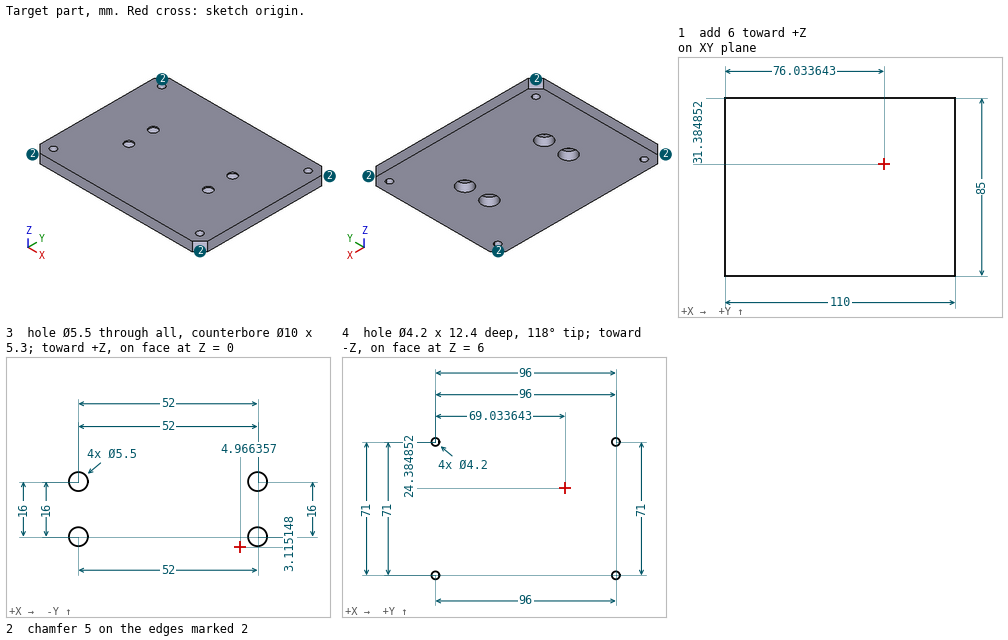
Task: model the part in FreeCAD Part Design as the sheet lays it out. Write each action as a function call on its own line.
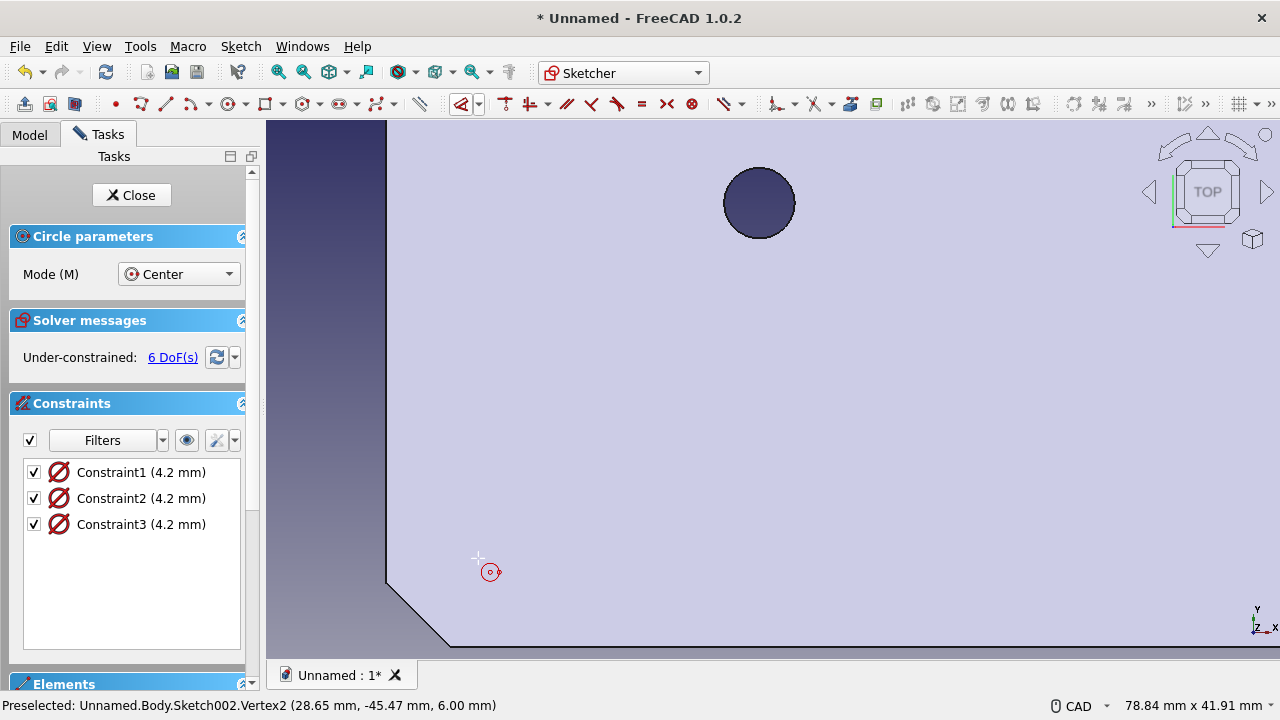
click(476, 557)
move(495, 538)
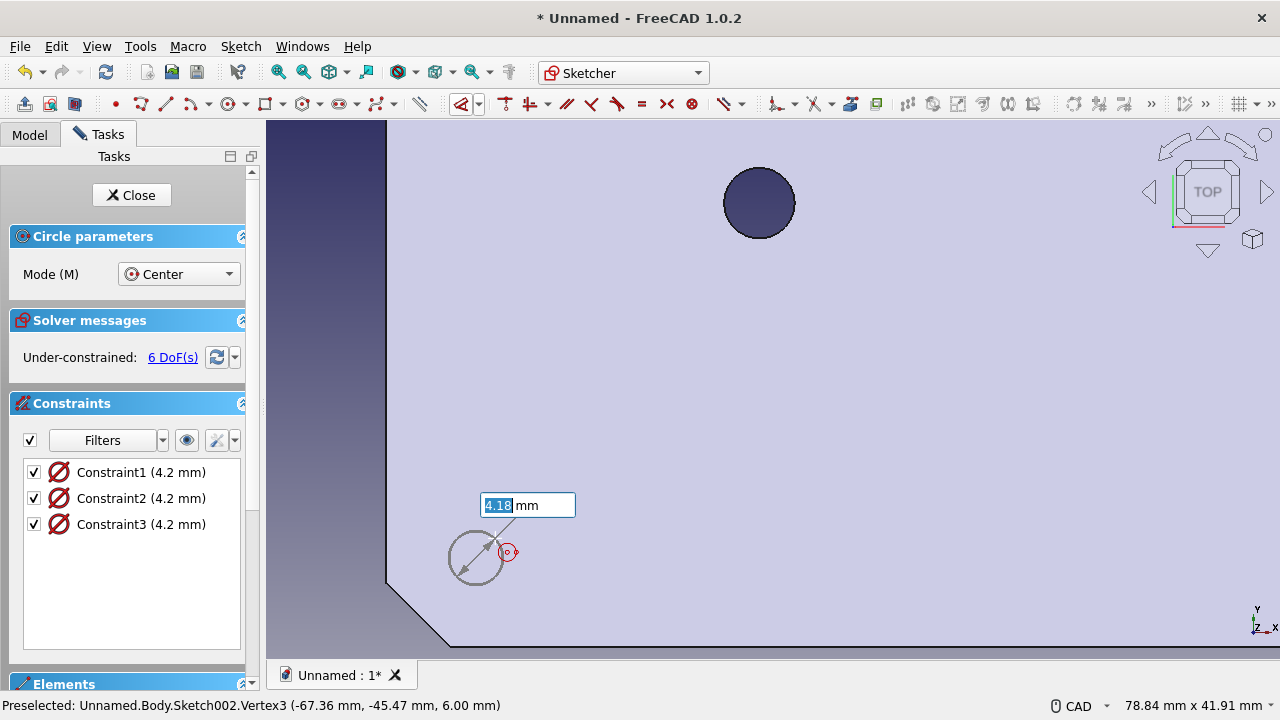
text(4.2)
key(Return)
key(Escape)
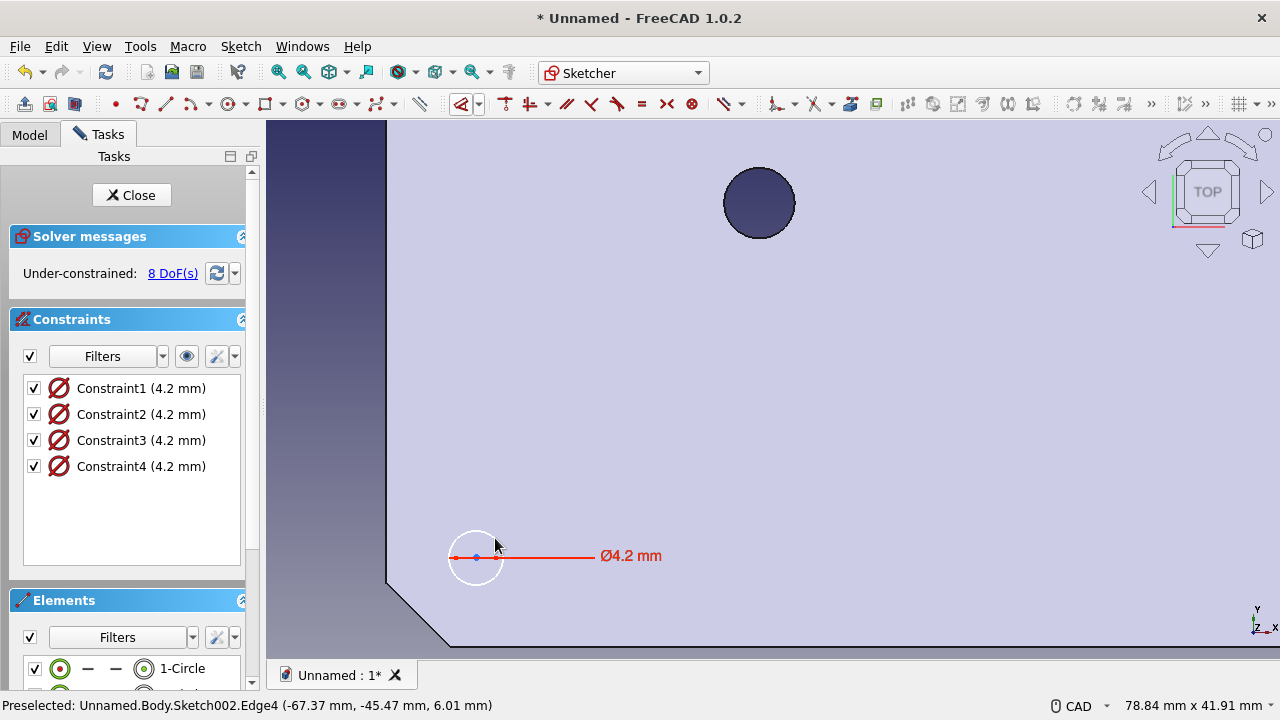
scroll(478, 558, down, 5)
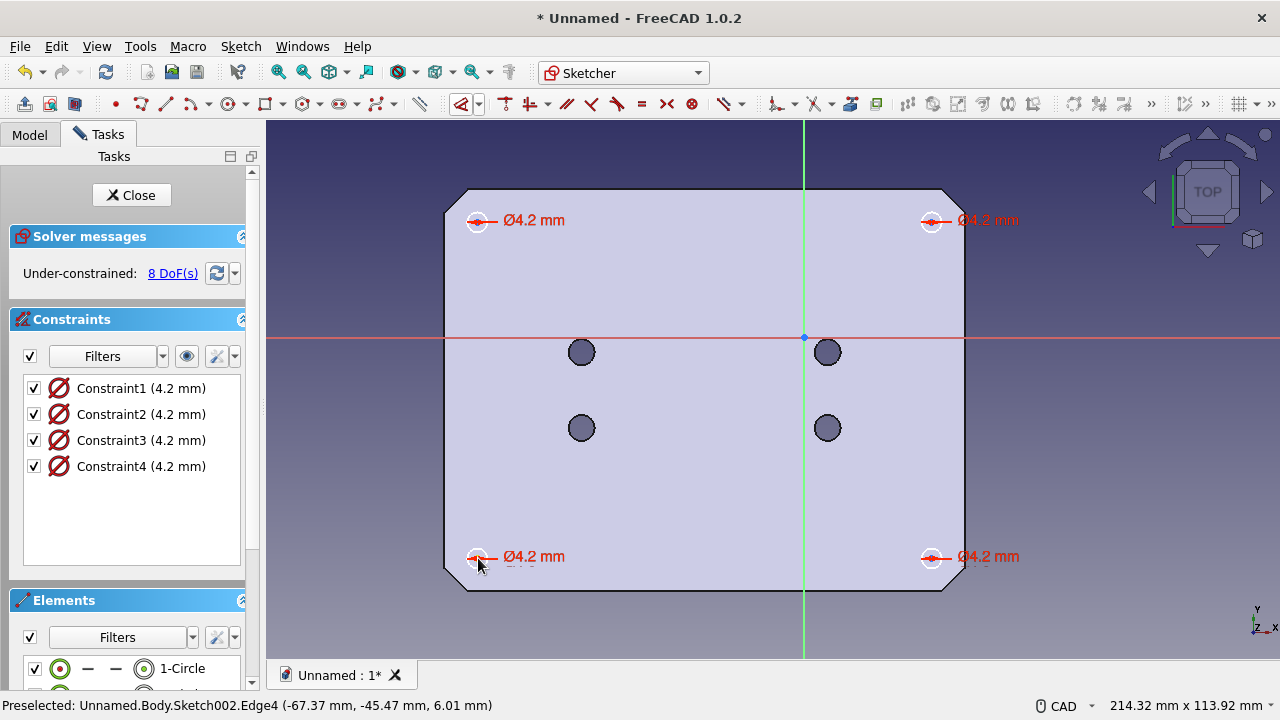
click(477, 222)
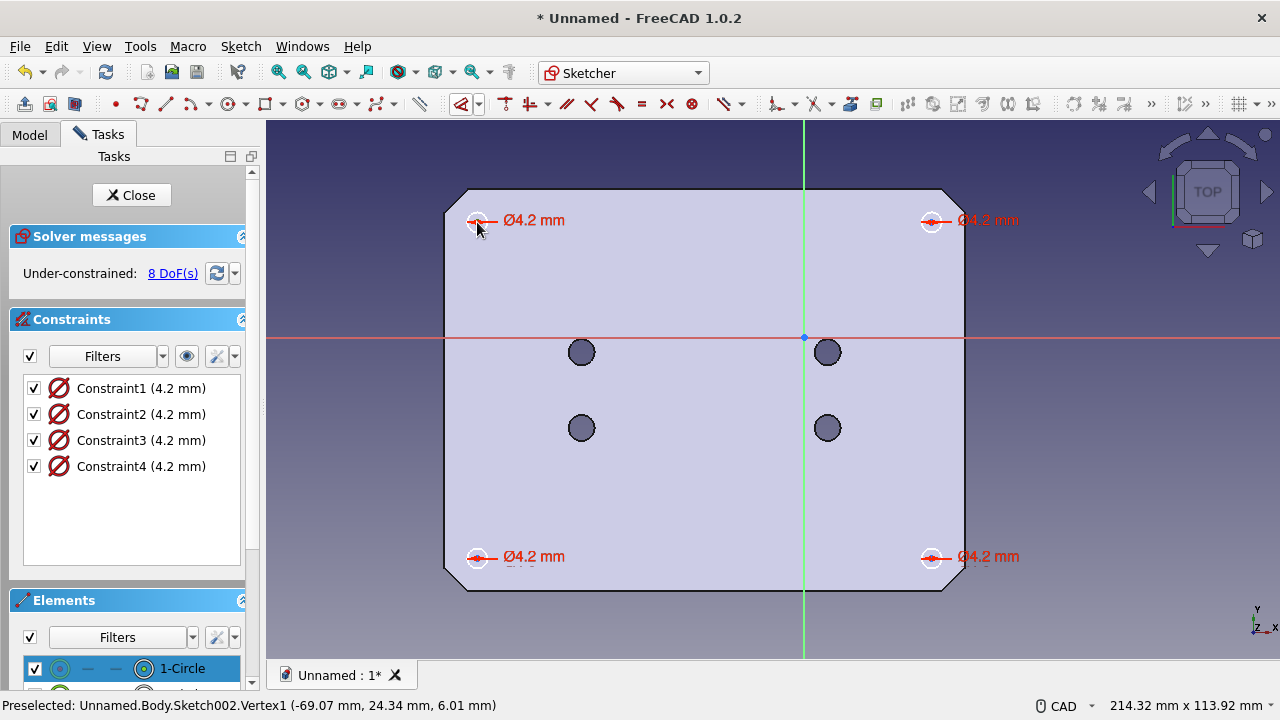
click(932, 222)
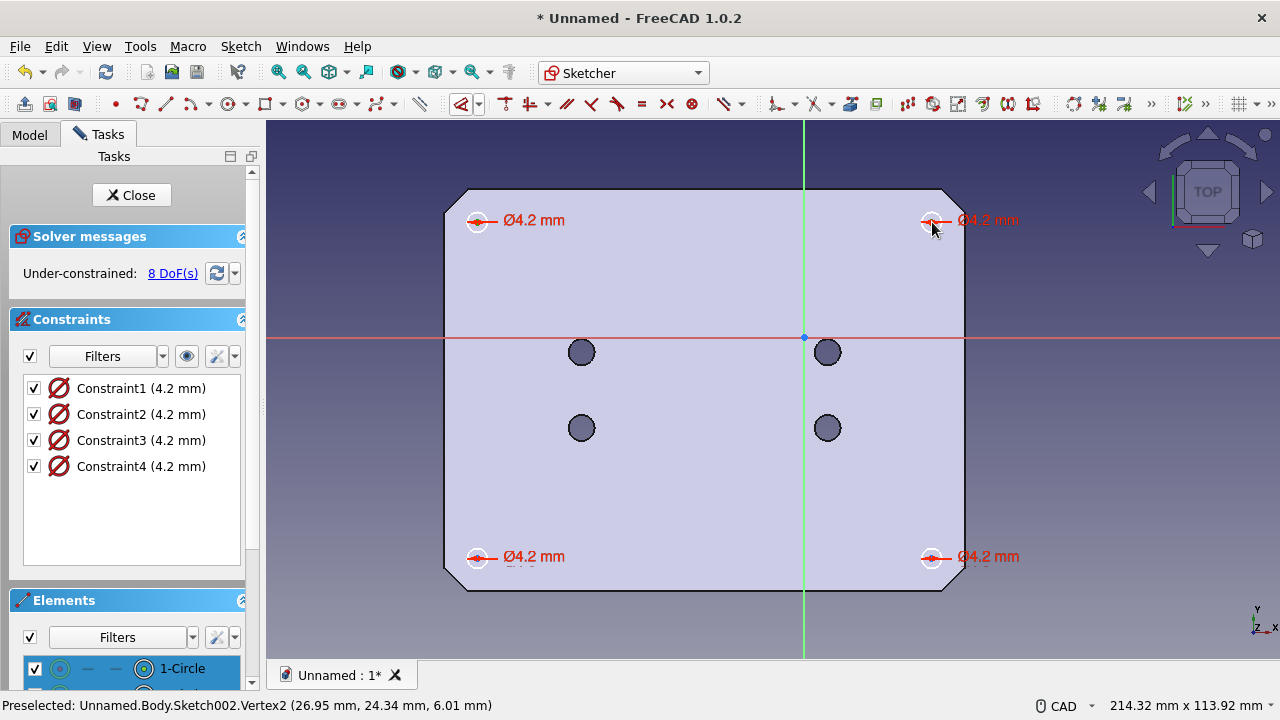
key(l)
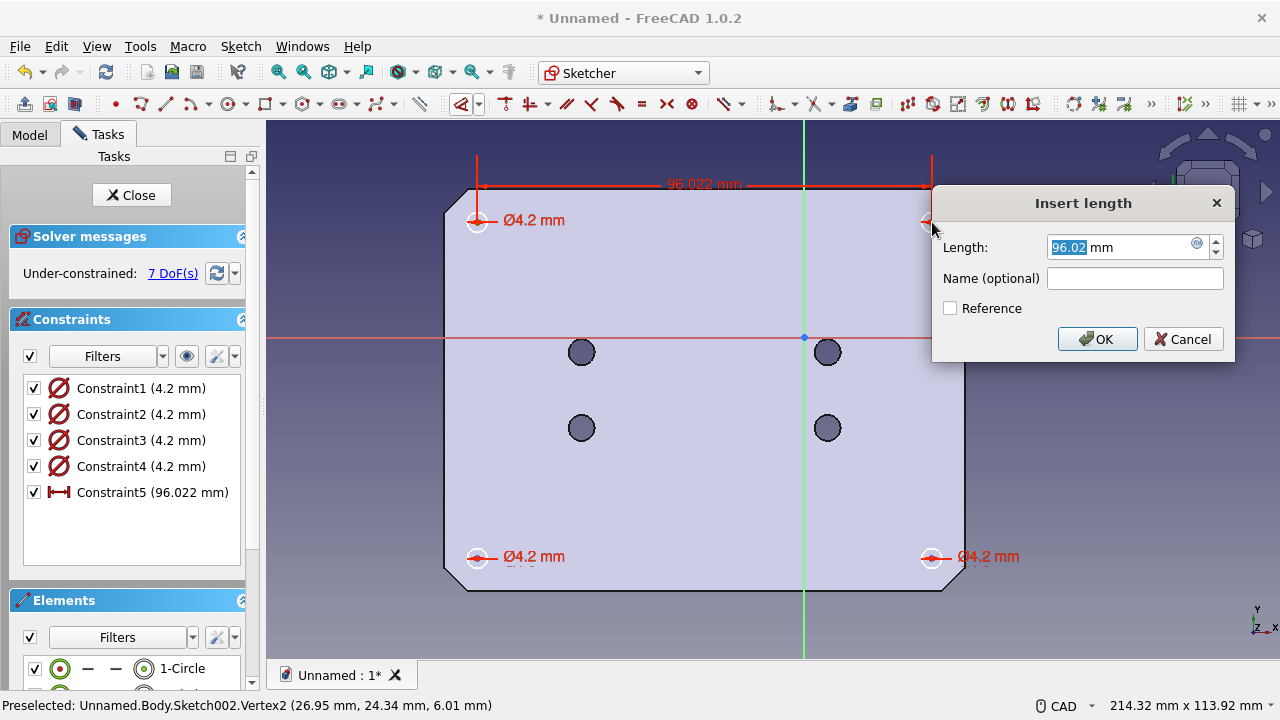
text(96)
key(Return)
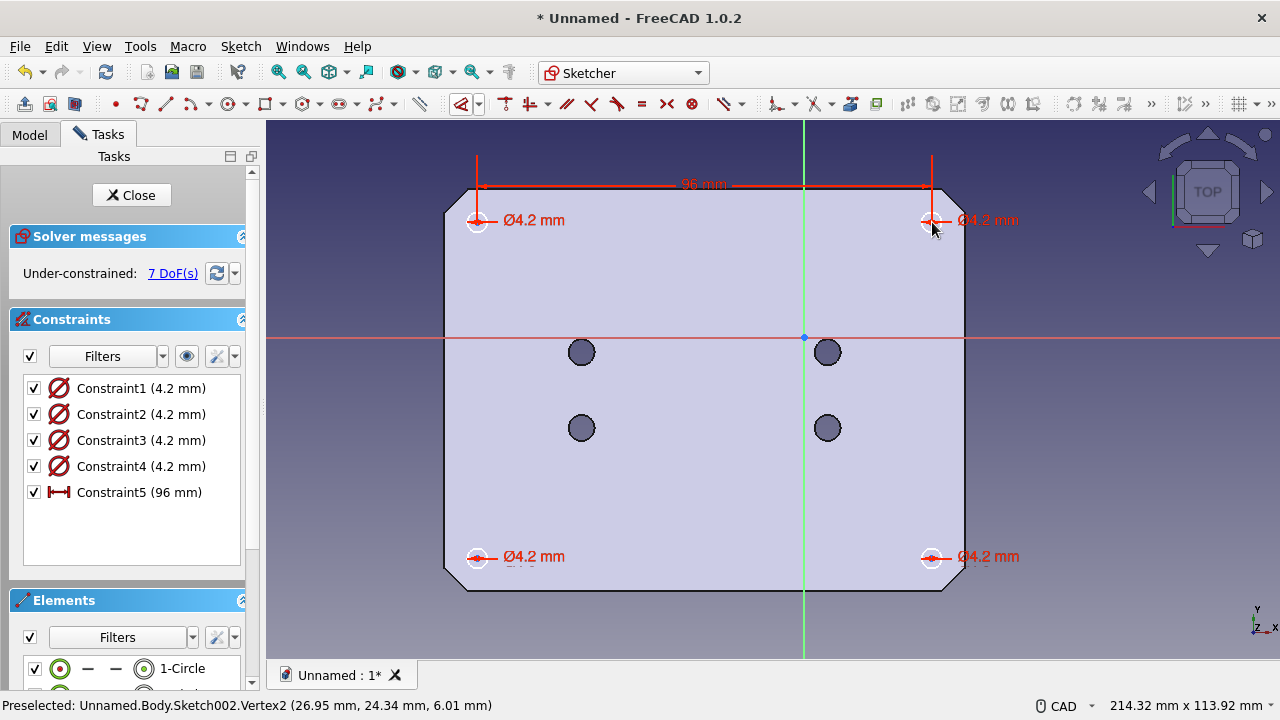
click(477, 222)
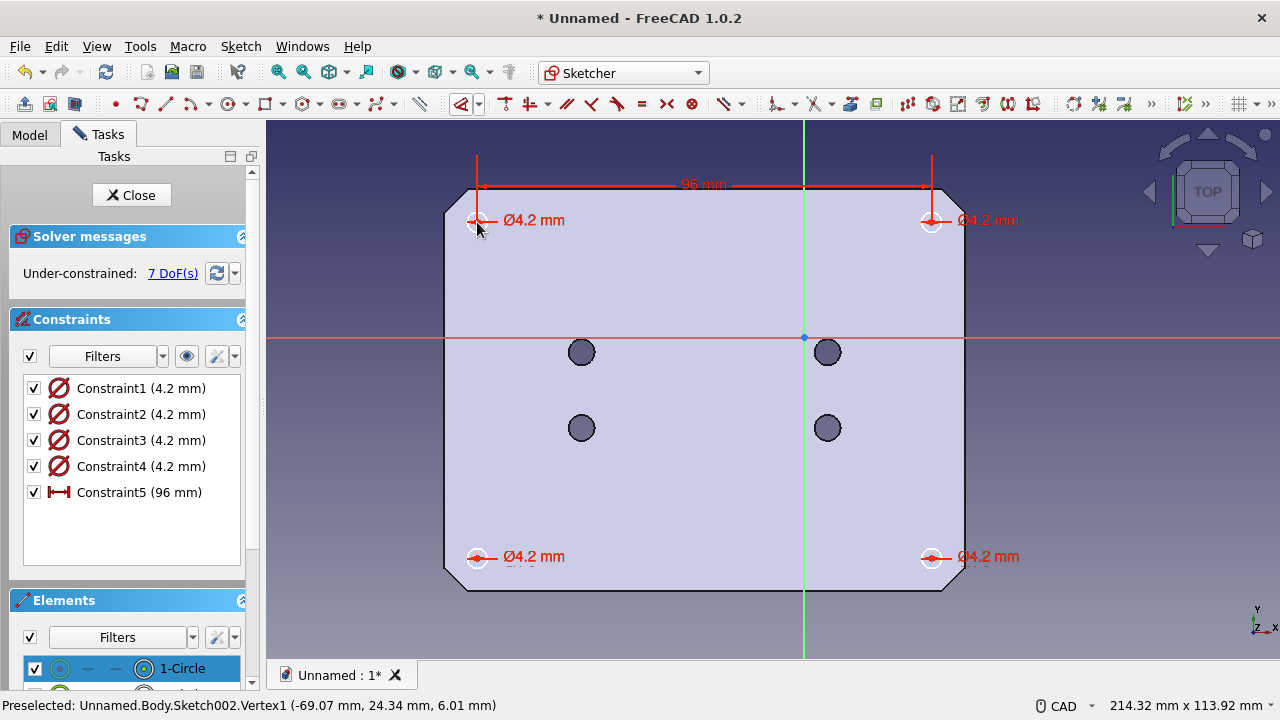
click(932, 559)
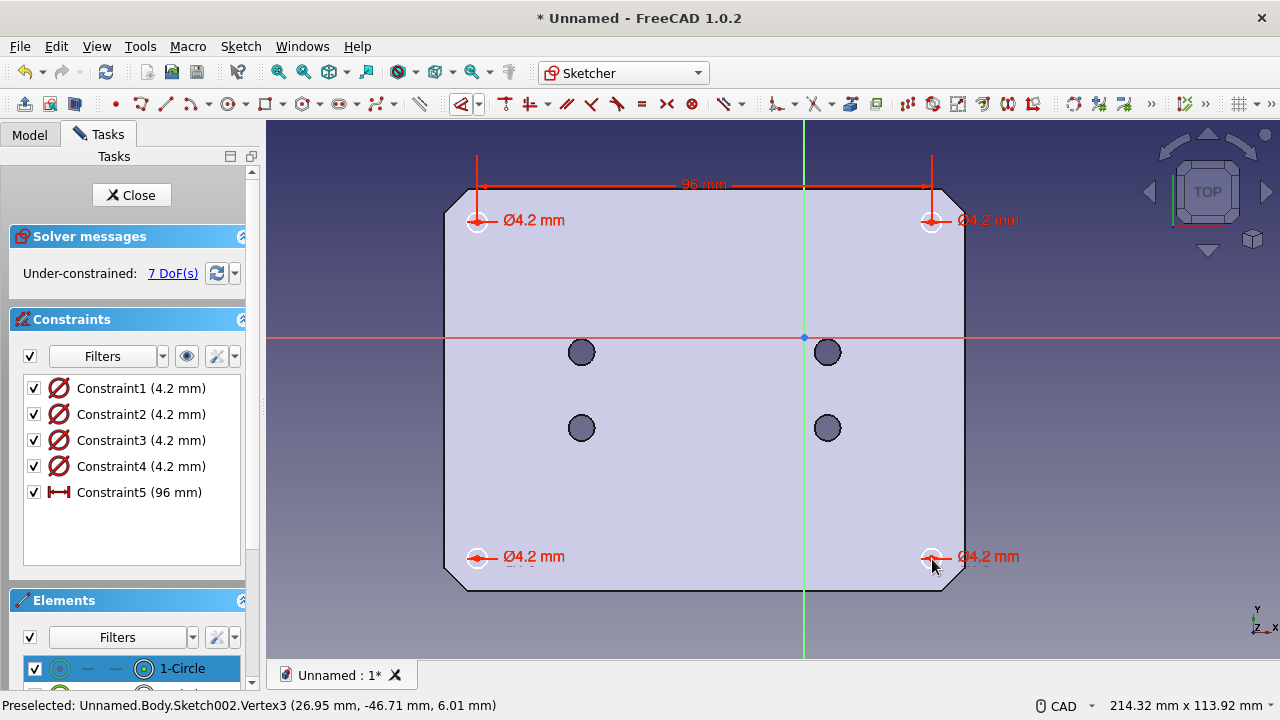
key(l)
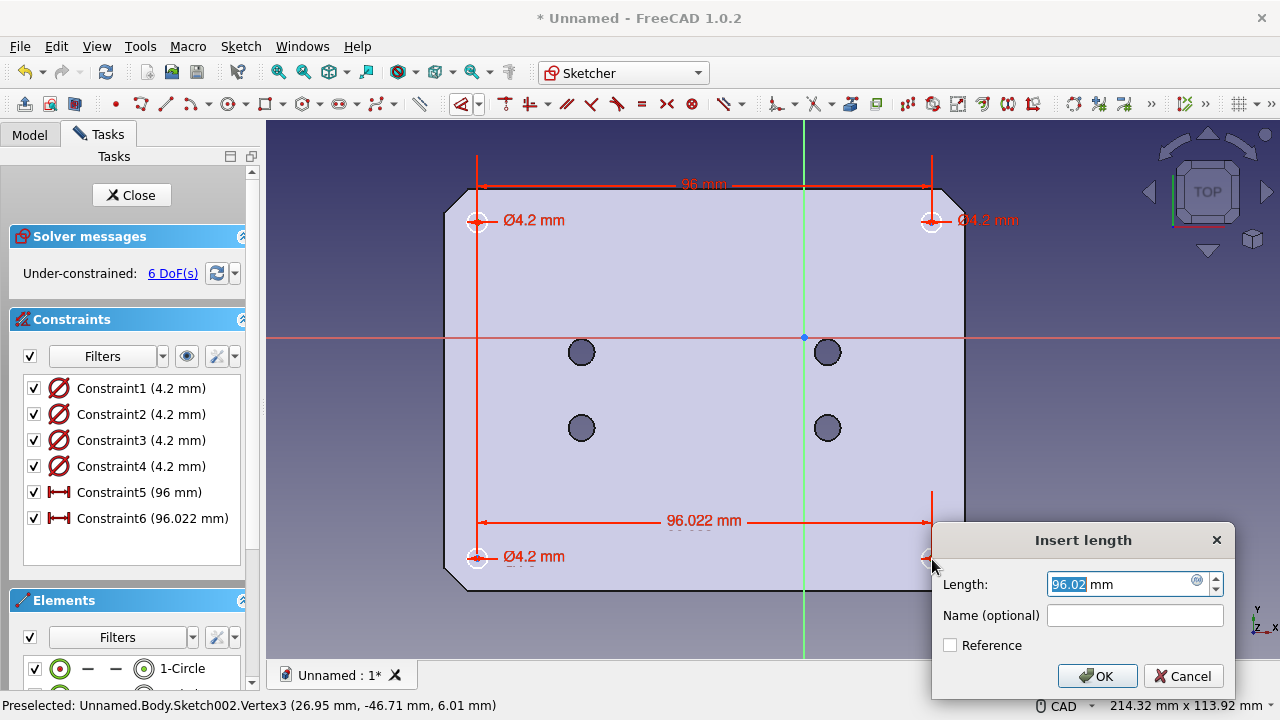
text(96)
key(Return)